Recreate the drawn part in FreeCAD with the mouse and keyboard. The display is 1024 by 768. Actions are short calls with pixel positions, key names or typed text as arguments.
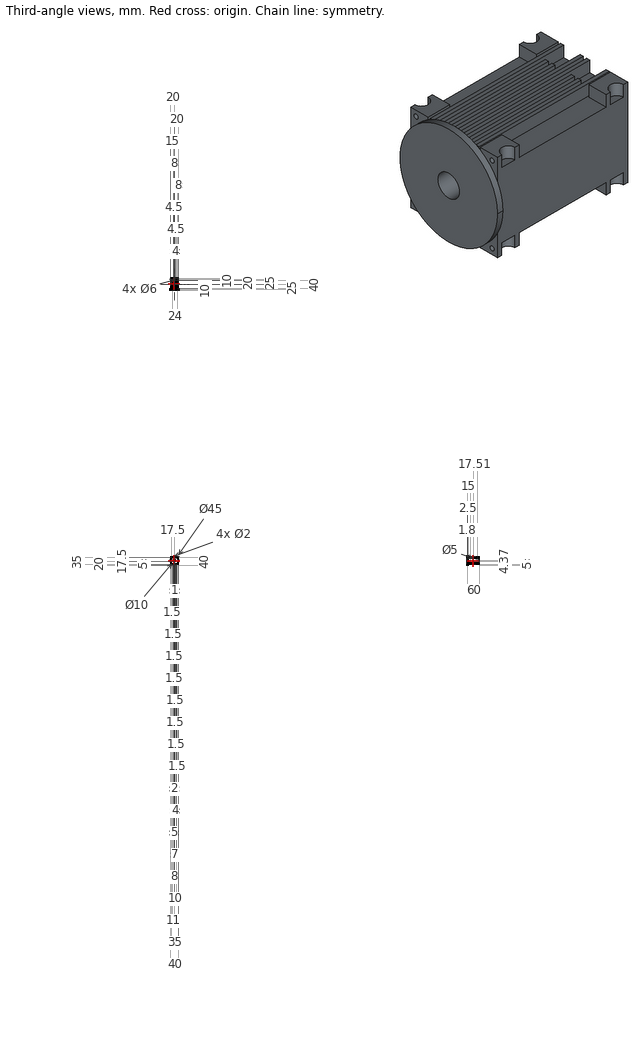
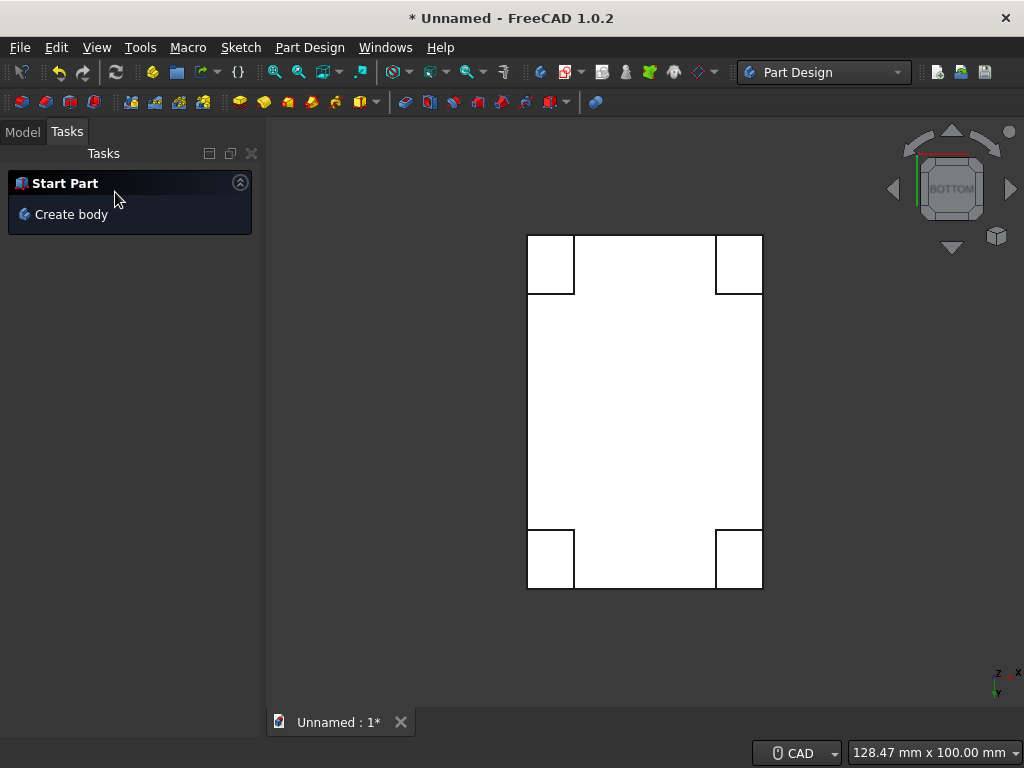
click(23, 131)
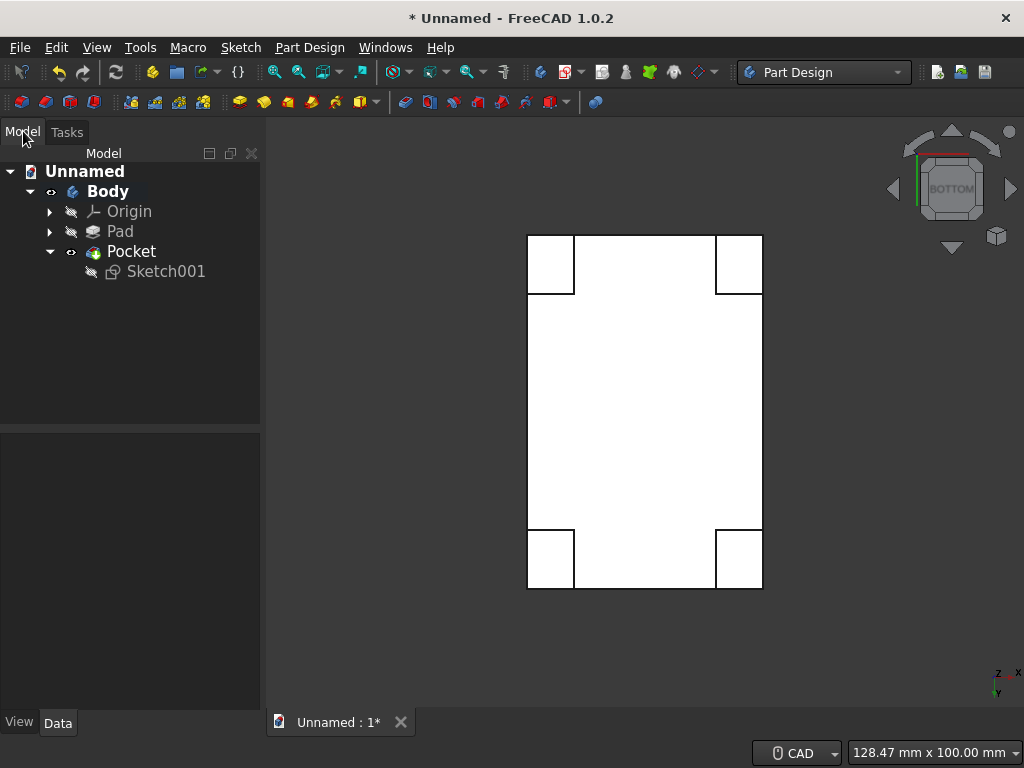
click(116, 252)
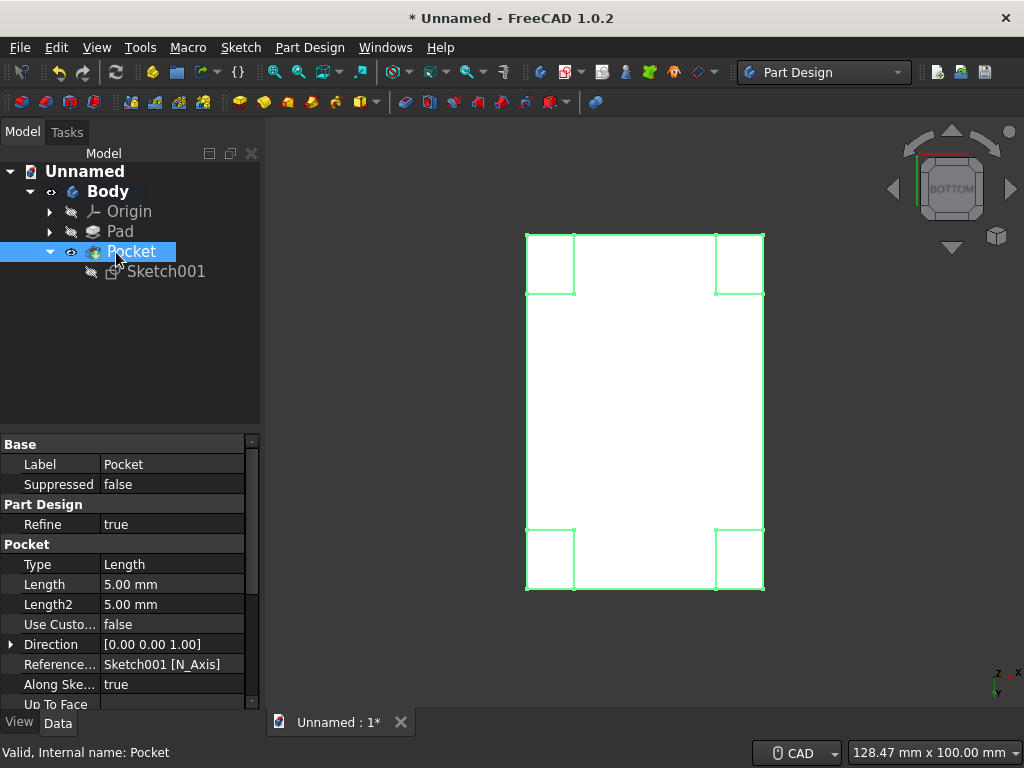
click(132, 102)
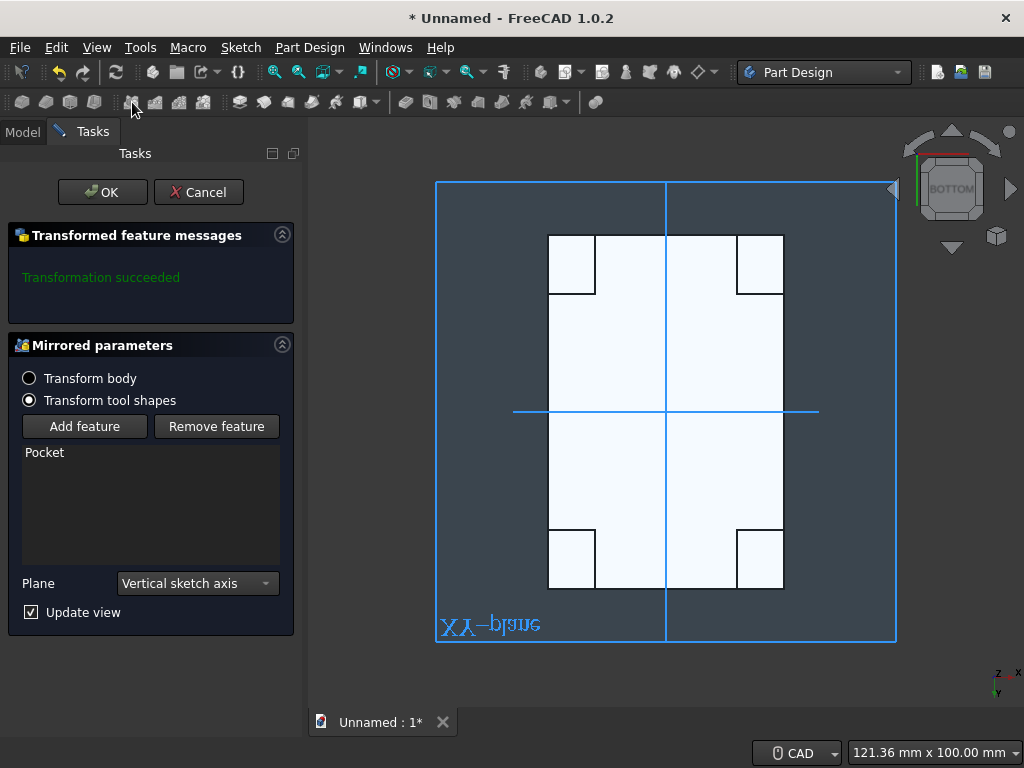
click(198, 584)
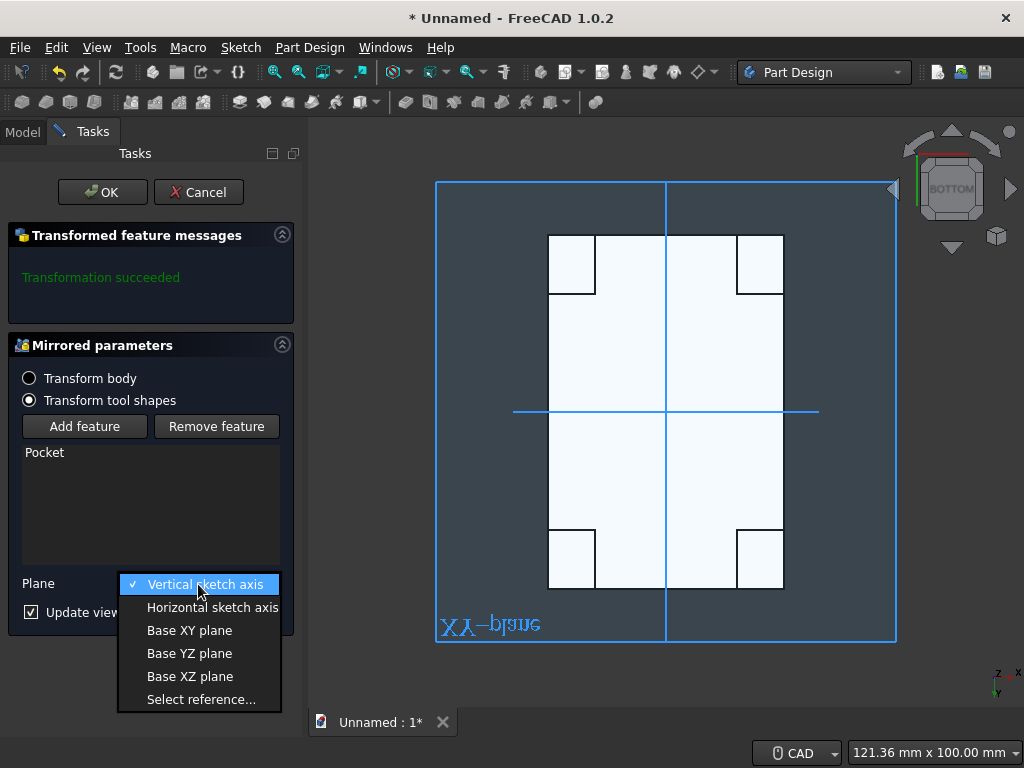
click(198, 630)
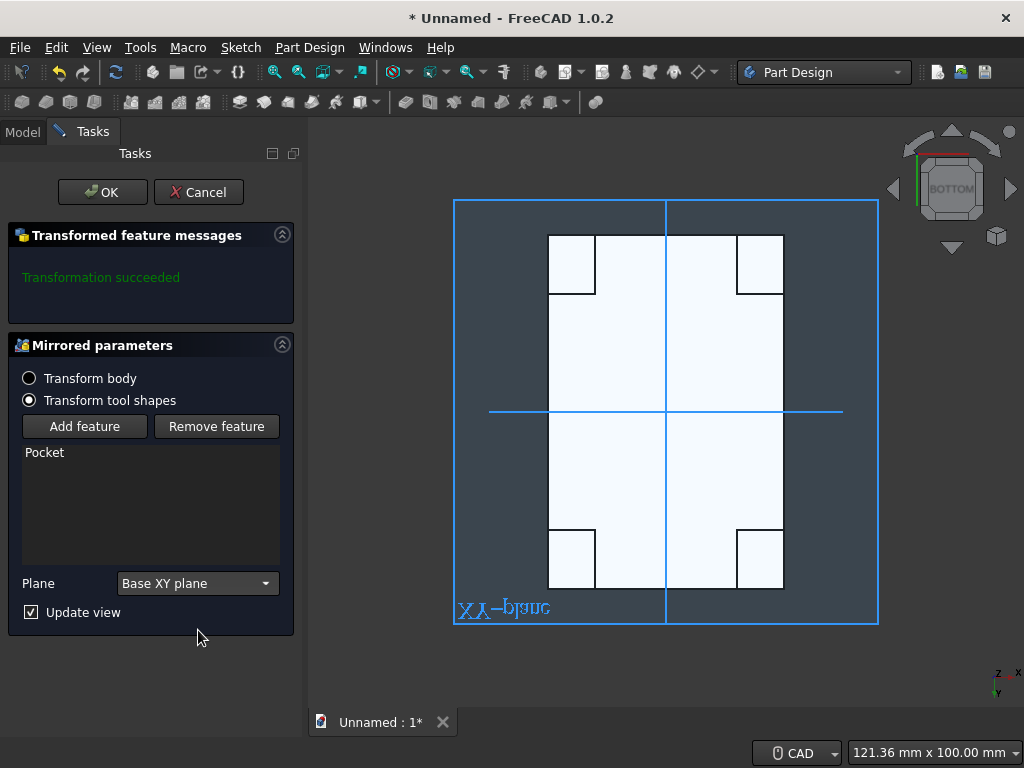
click(103, 192)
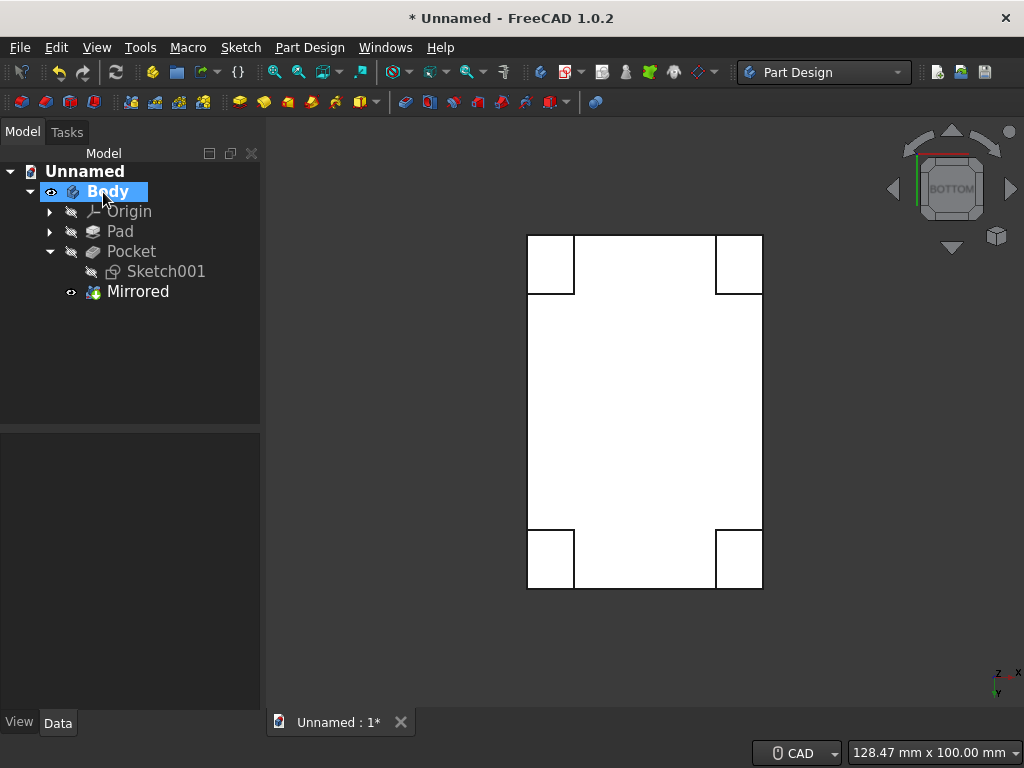
key(4)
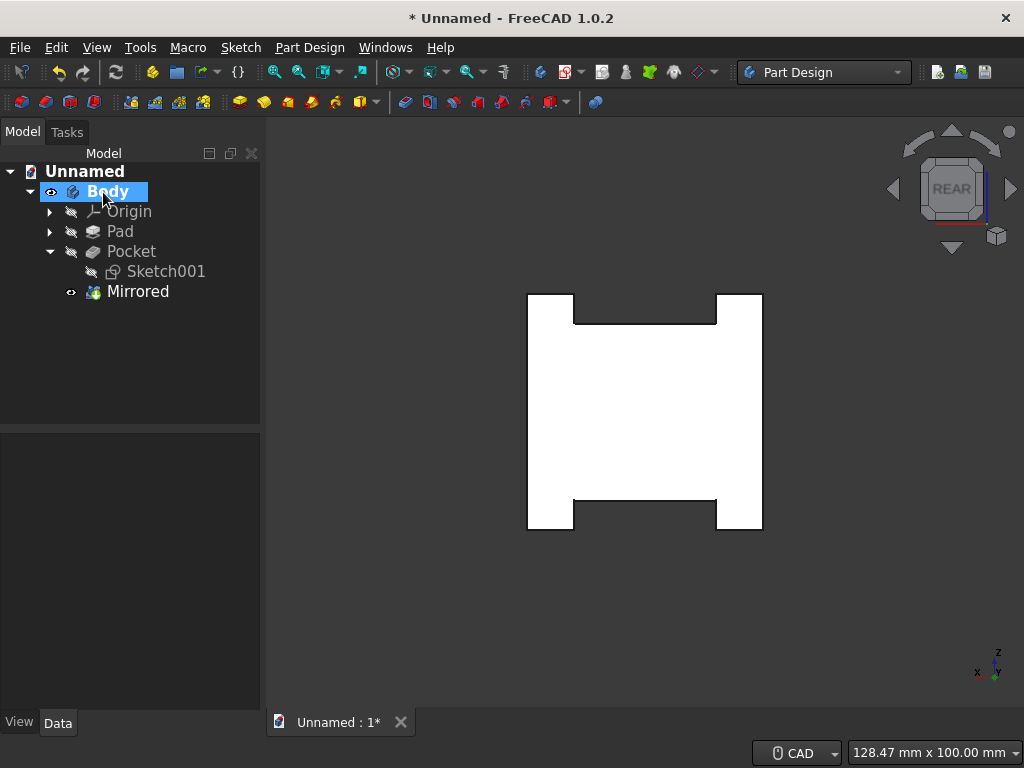
click(276, 72)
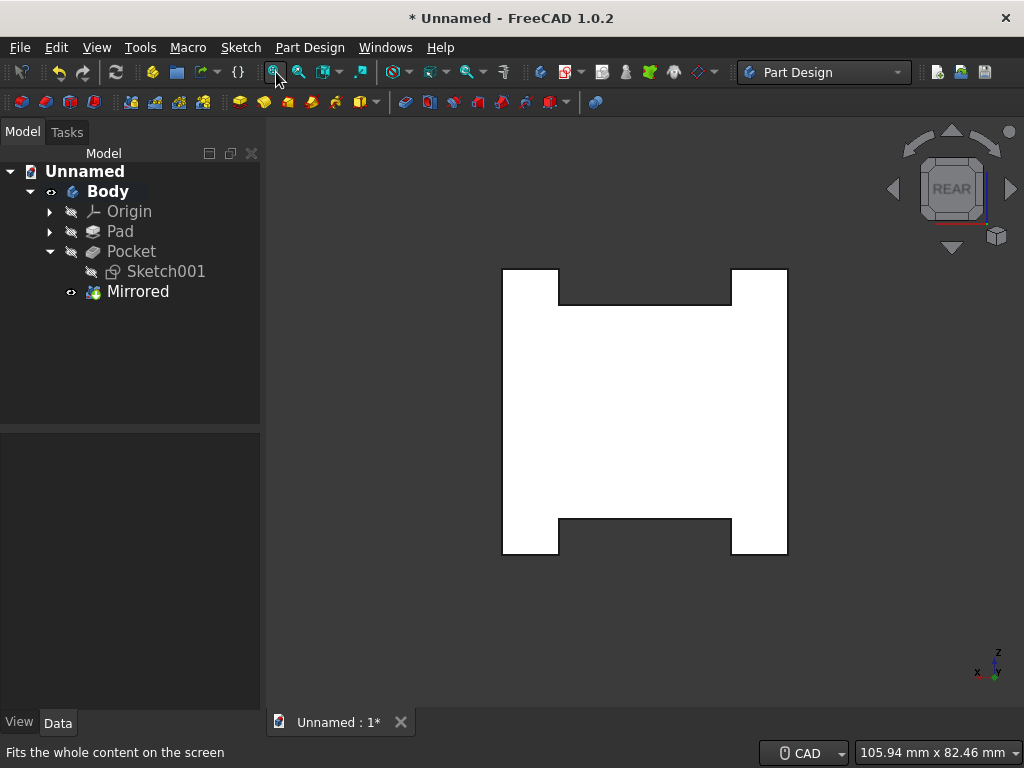
click(645, 411)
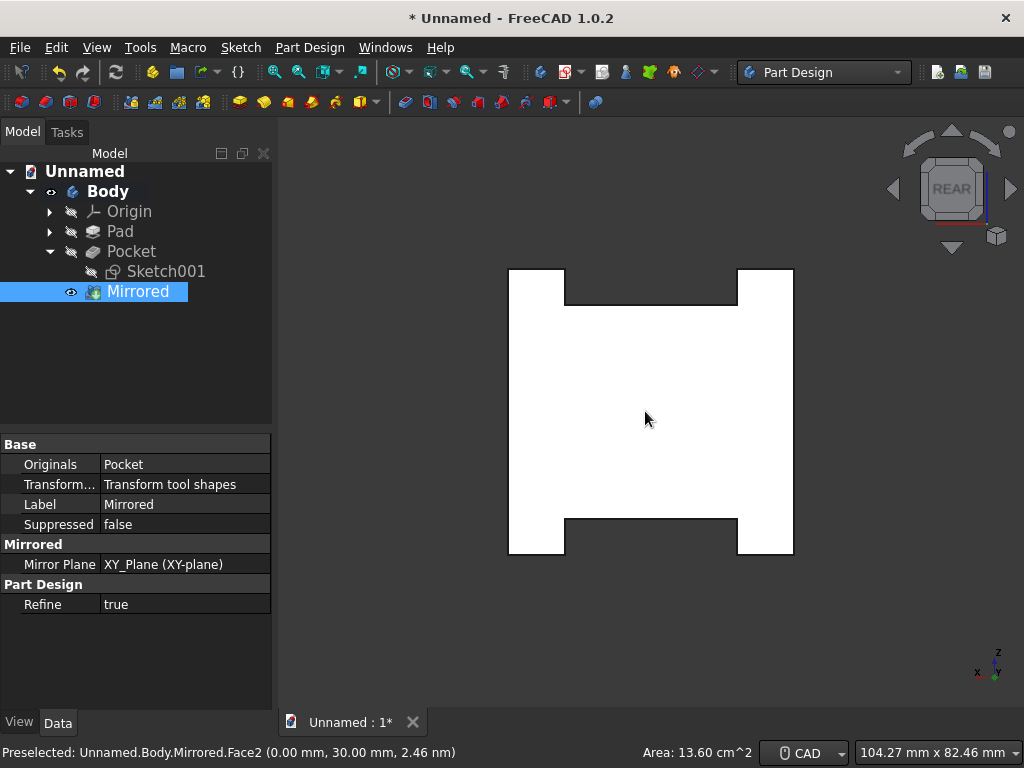
click(566, 72)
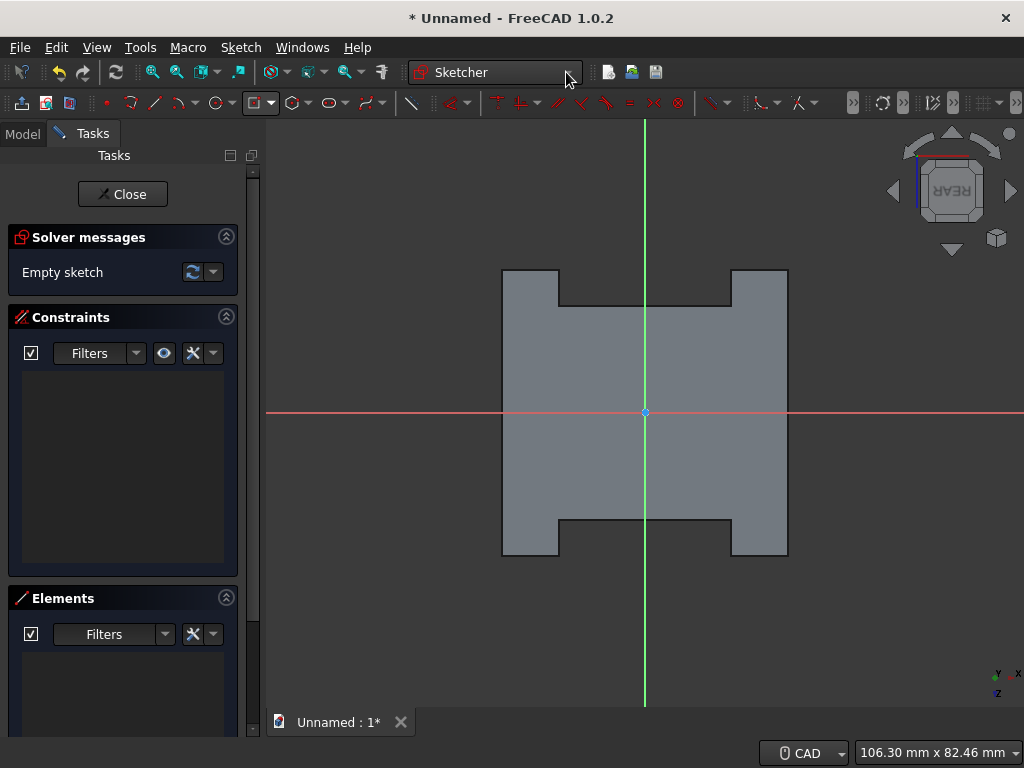
scroll(688, 300, up, 5)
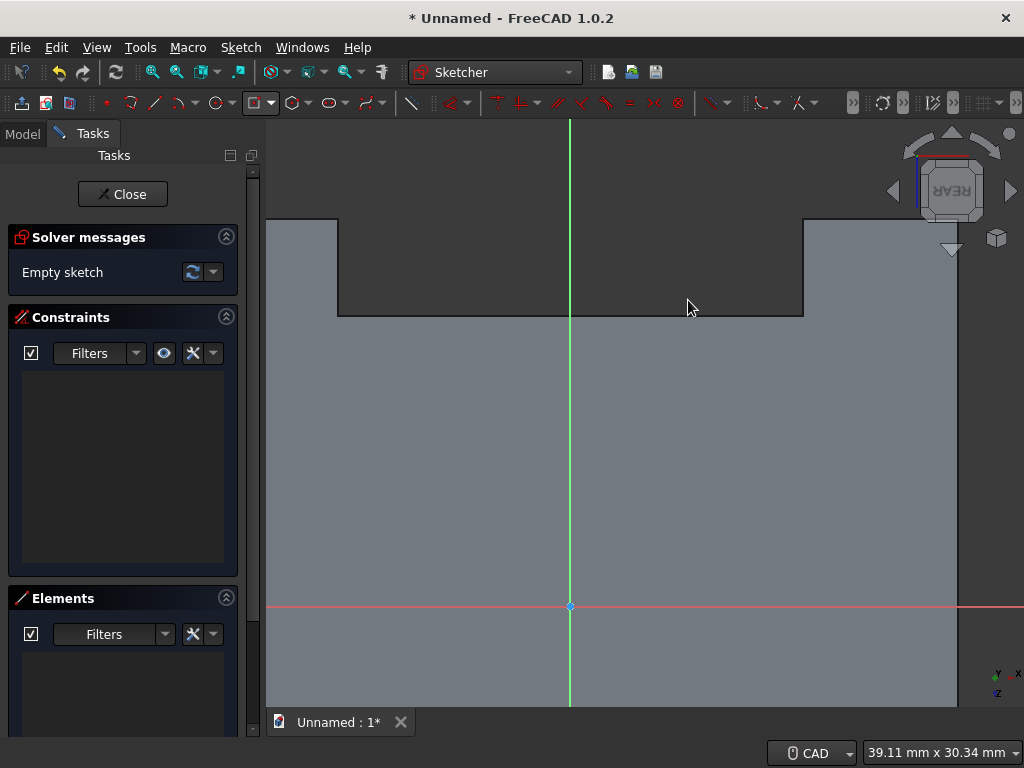
click(274, 104)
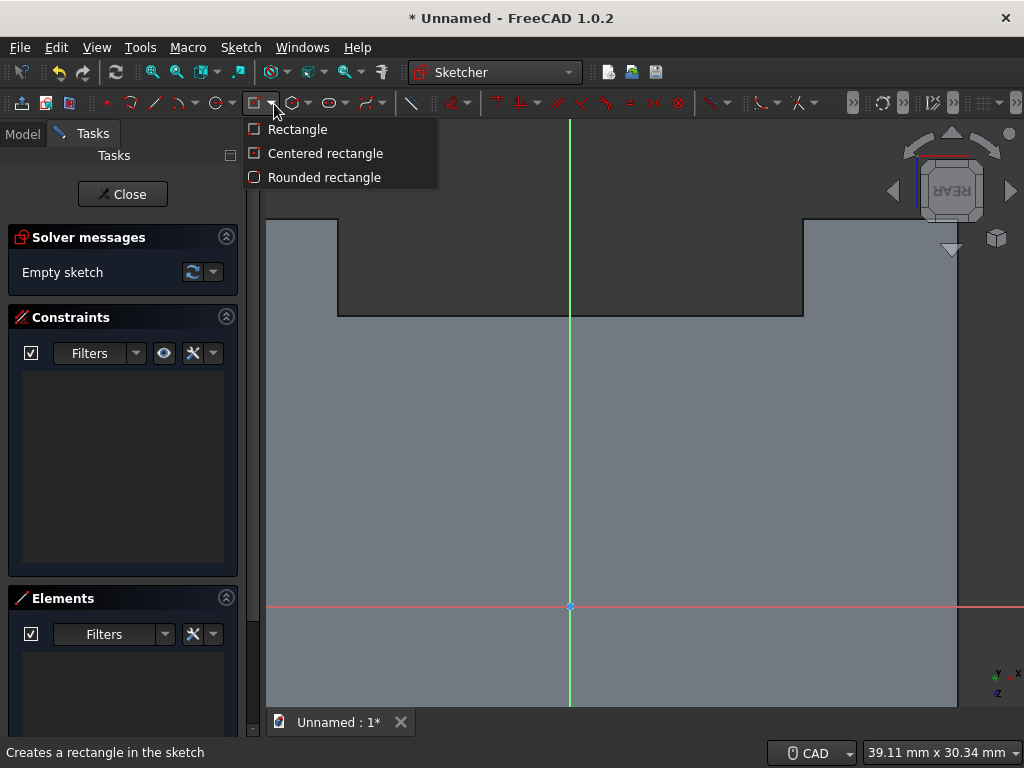
click(340, 129)